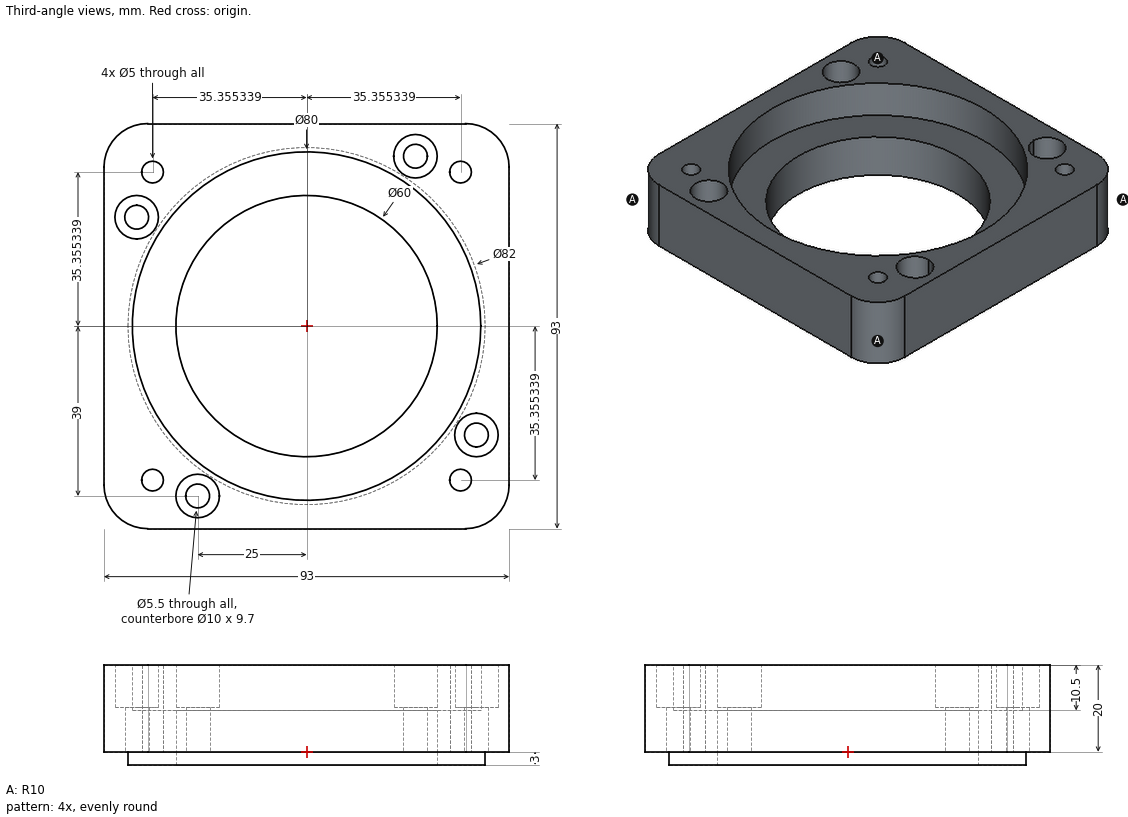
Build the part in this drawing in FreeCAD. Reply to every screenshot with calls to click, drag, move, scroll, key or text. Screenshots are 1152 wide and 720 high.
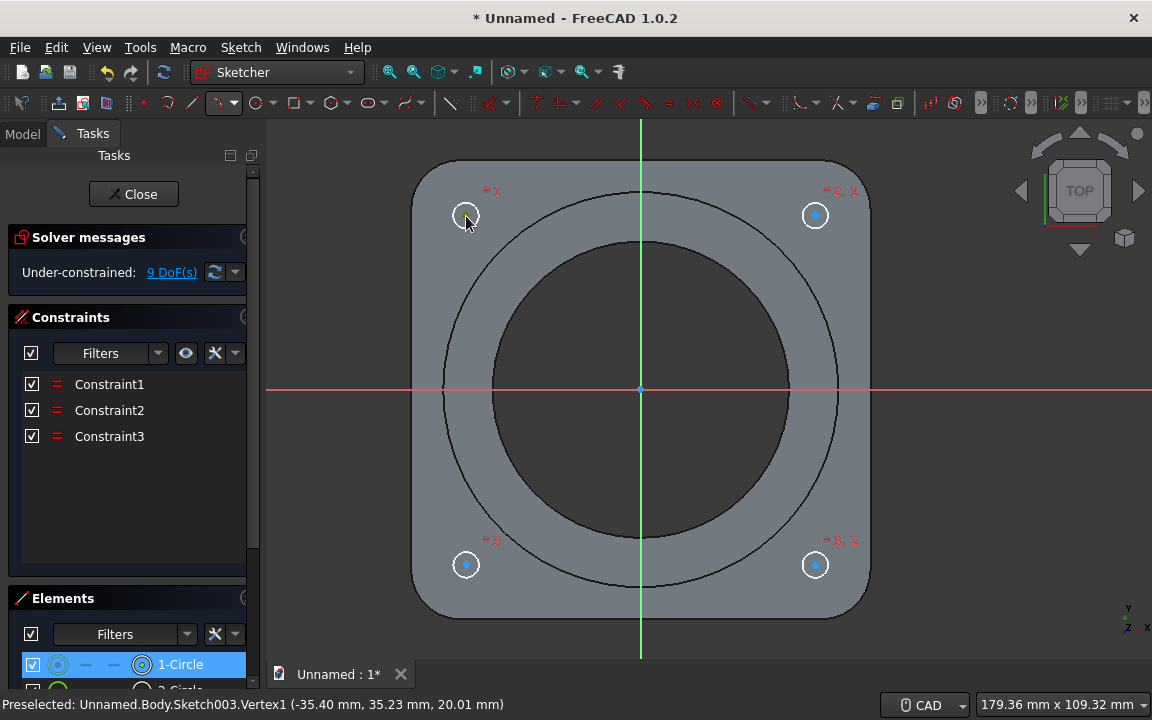
click(815, 216)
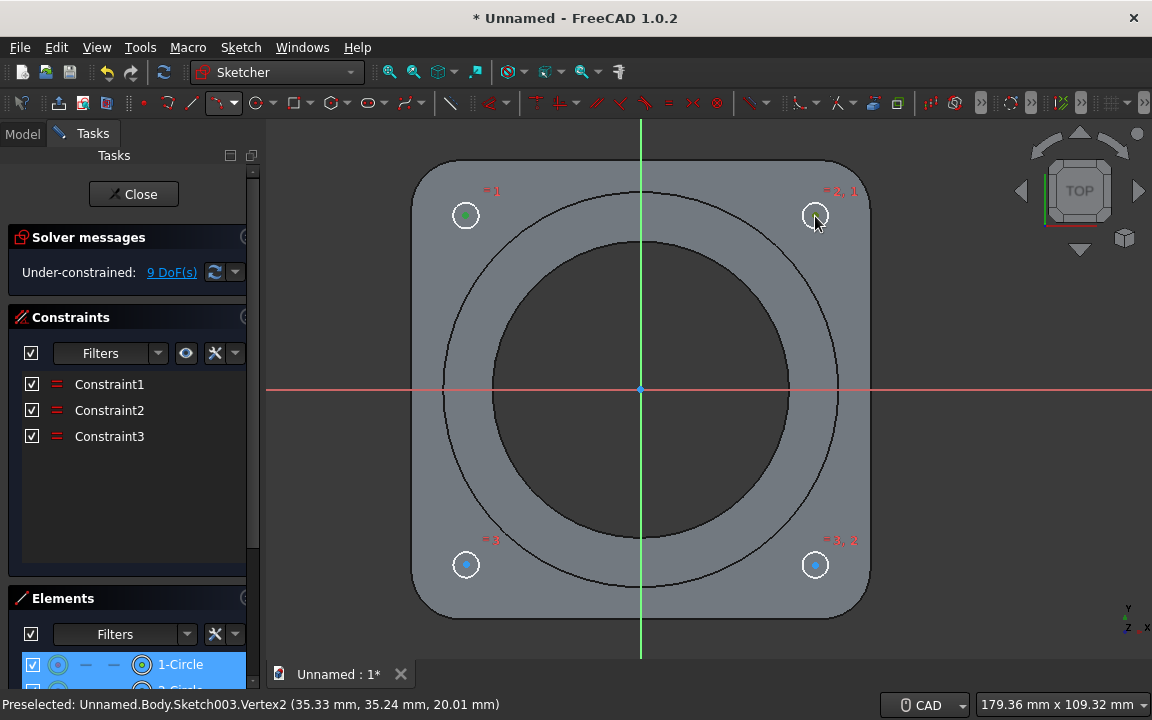
click(578, 104)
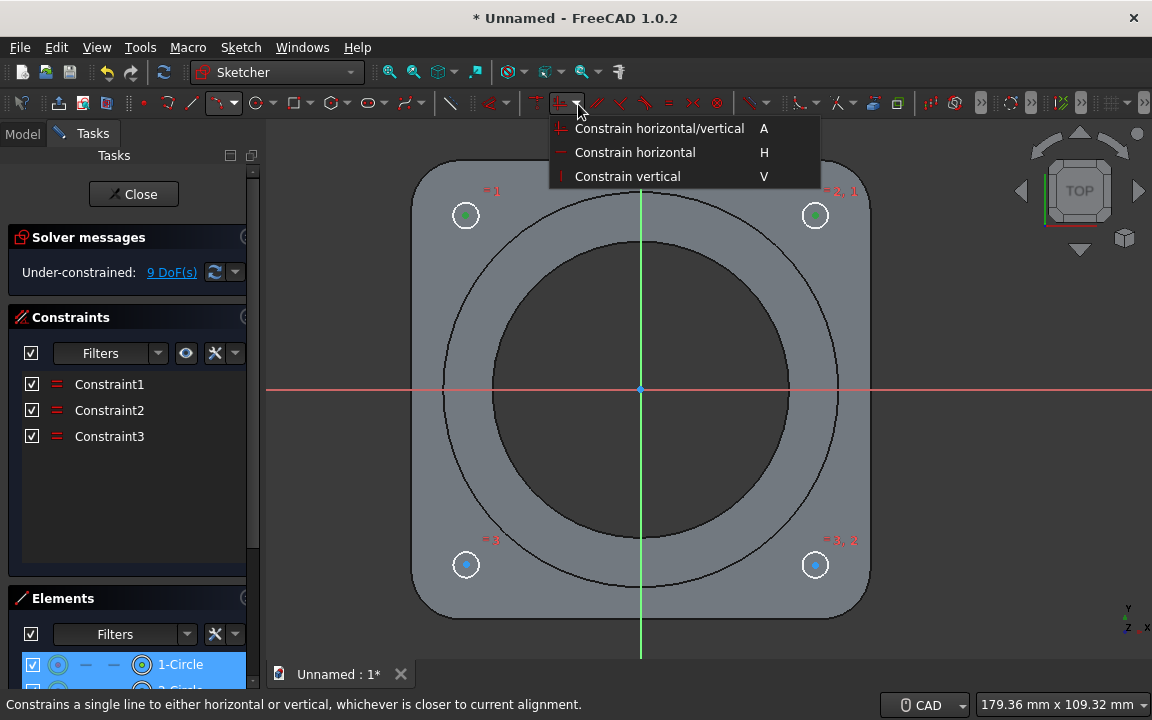
click(685, 152)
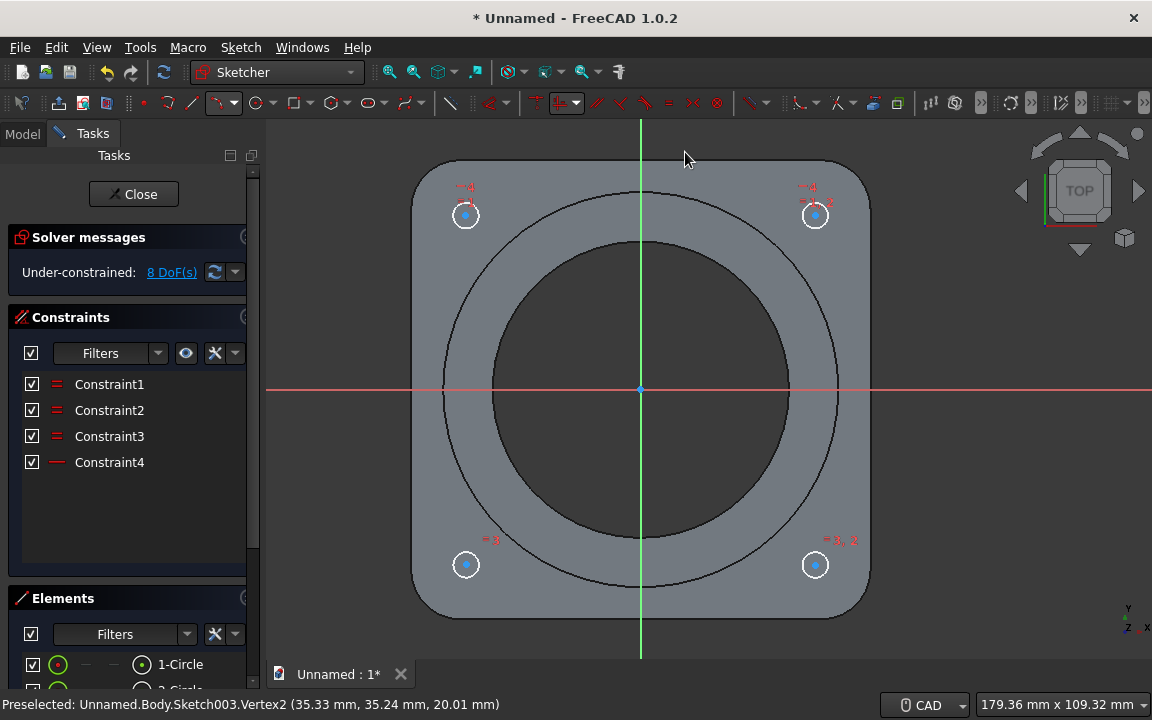
click(815, 216)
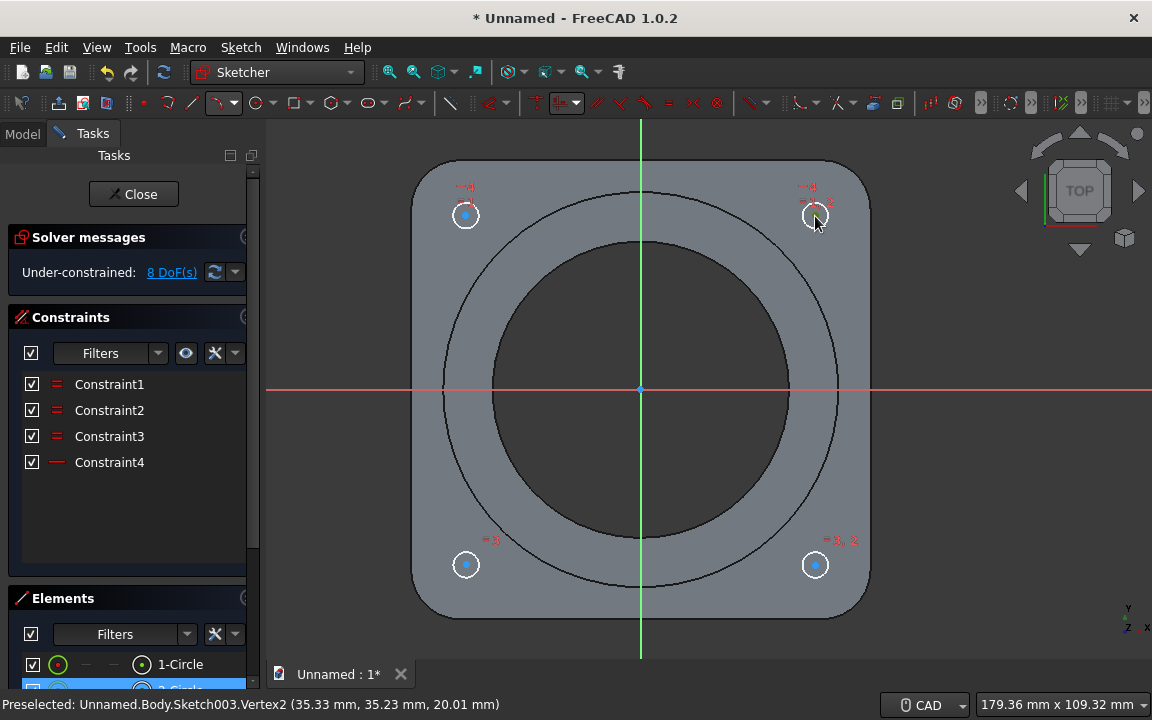
click(815, 565)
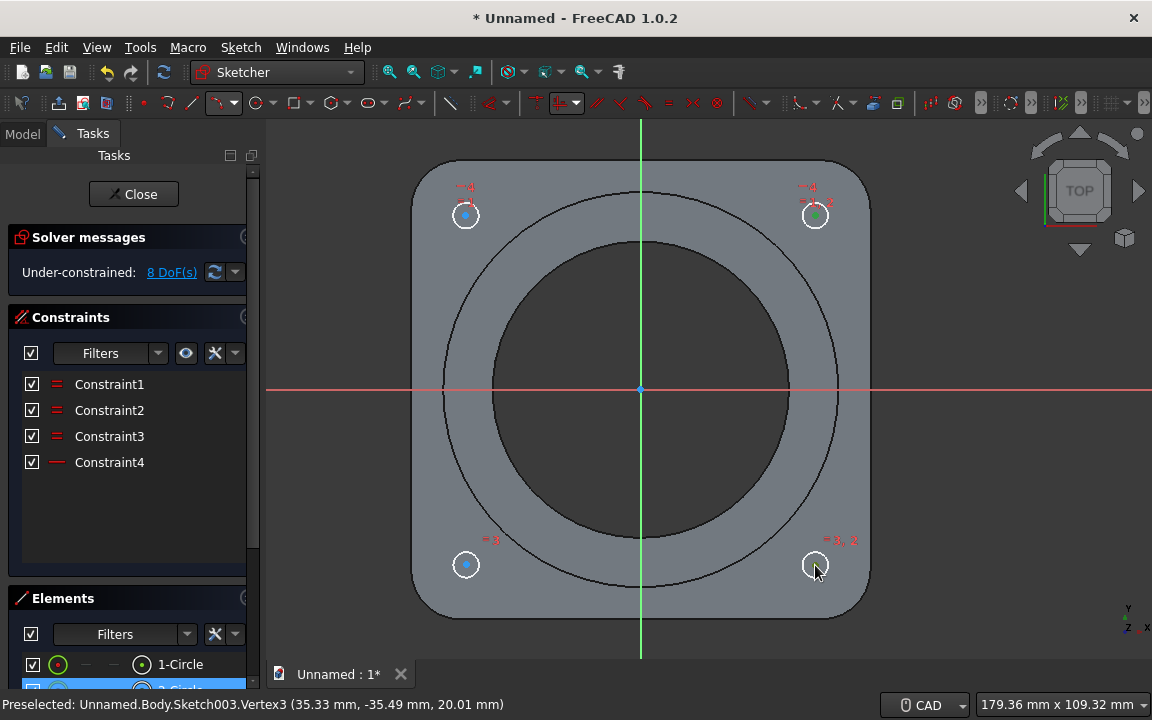
click(578, 104)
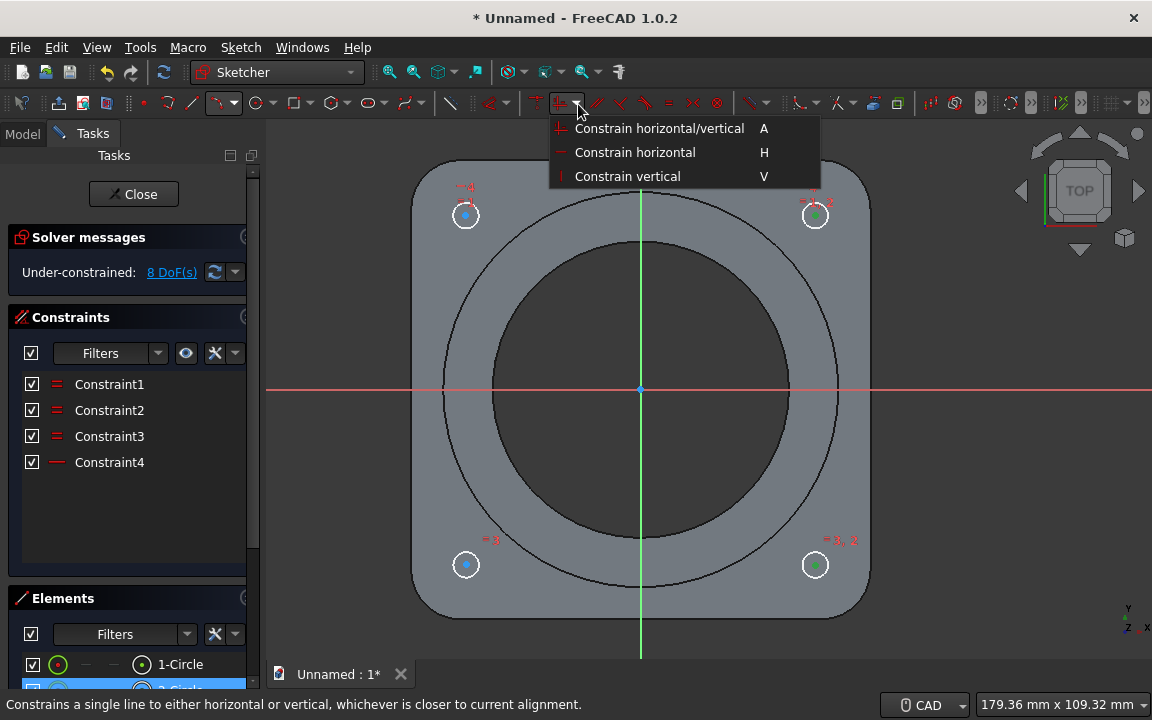
click(685, 176)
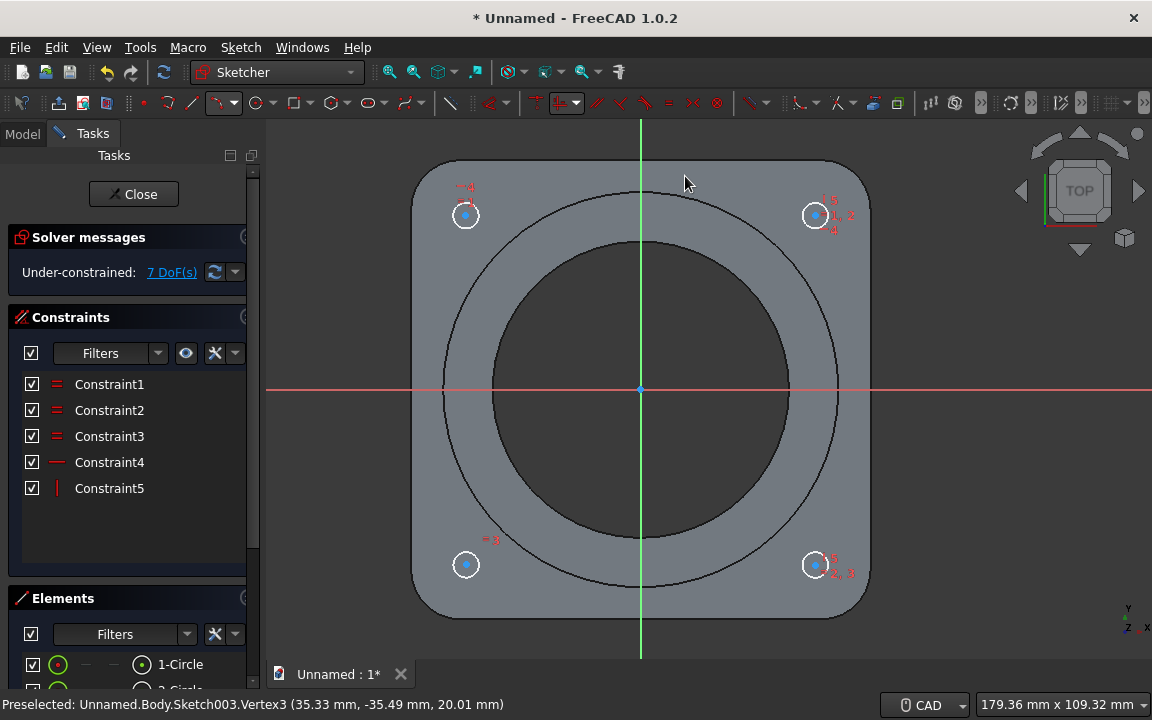
click(466, 216)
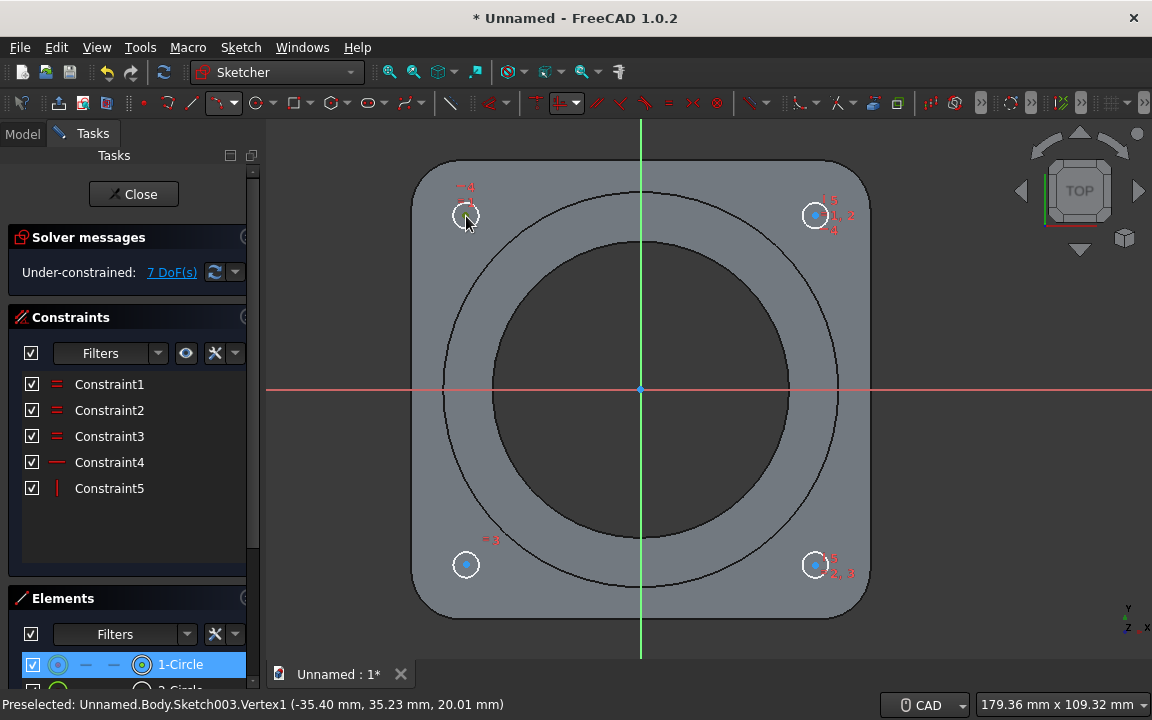
click(466, 565)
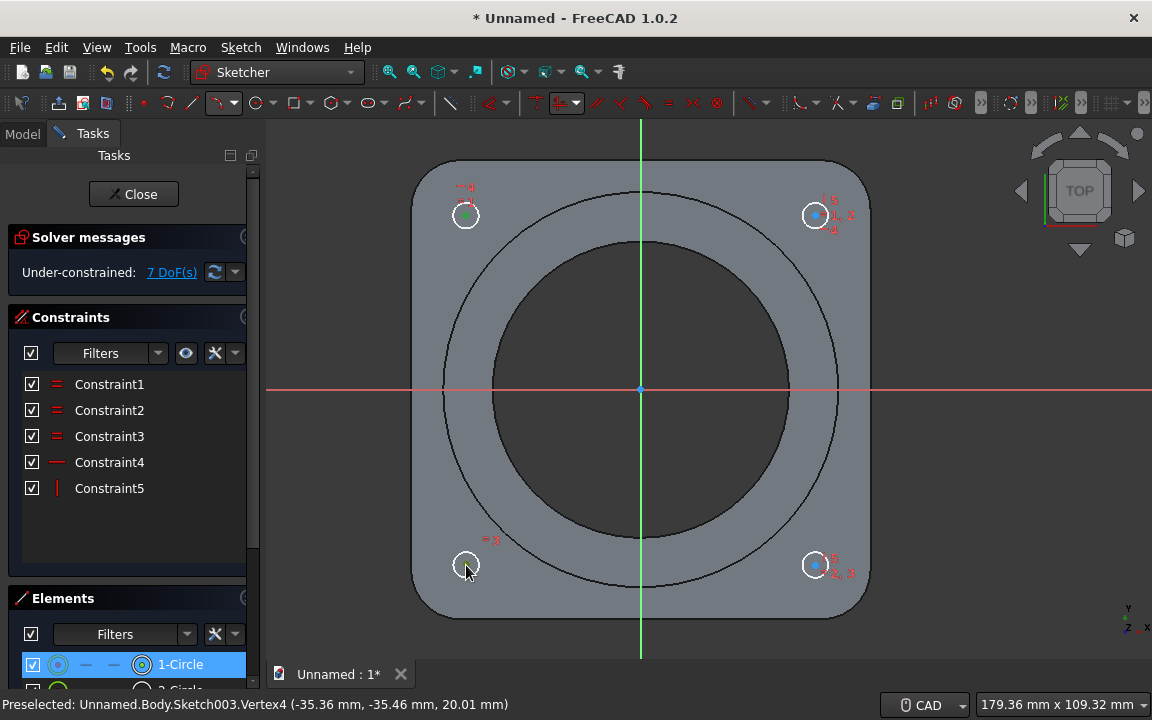
click(578, 104)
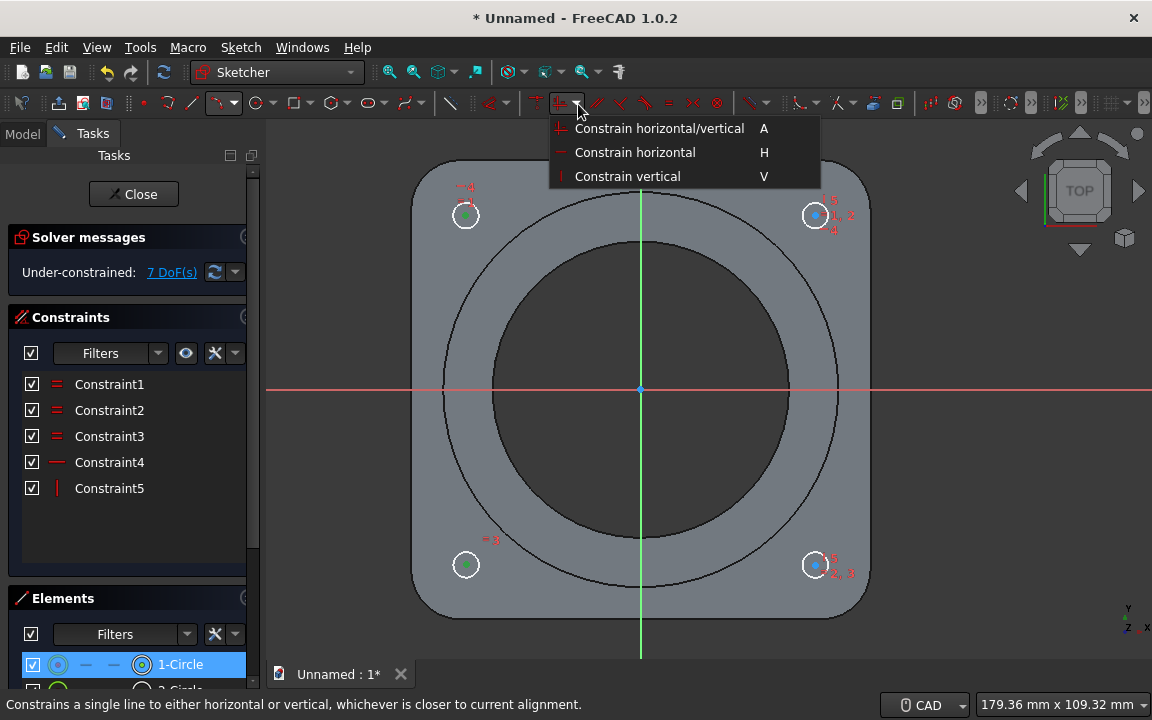
click(685, 176)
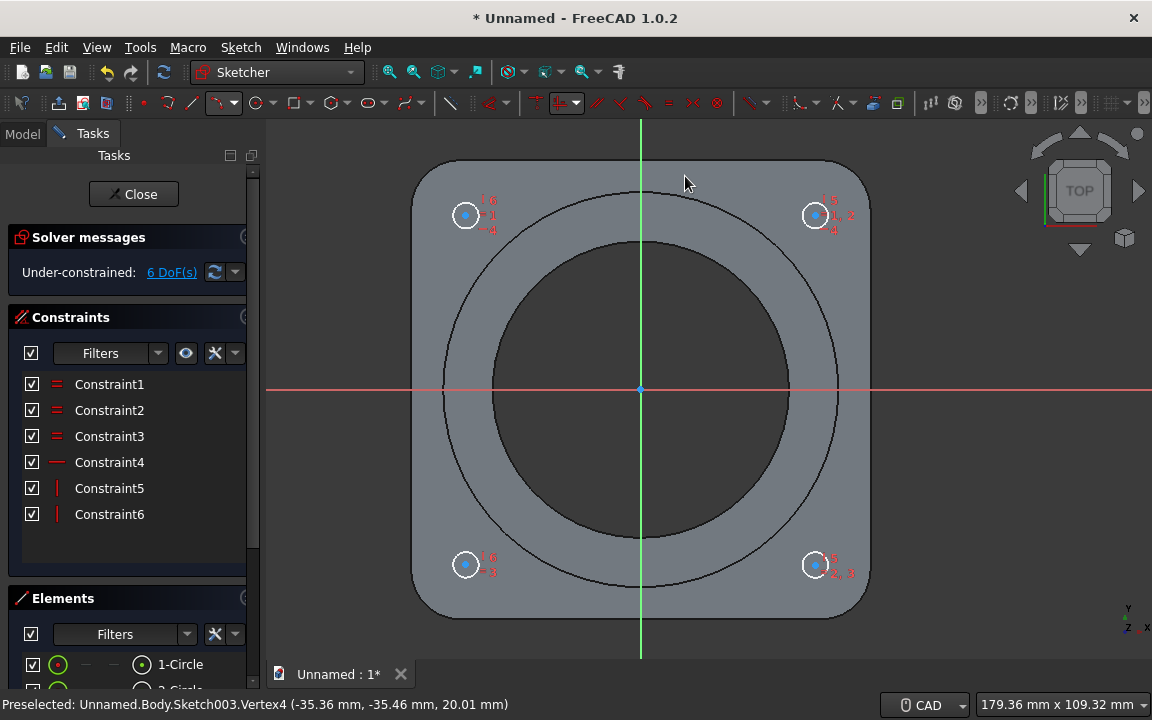
click(815, 565)